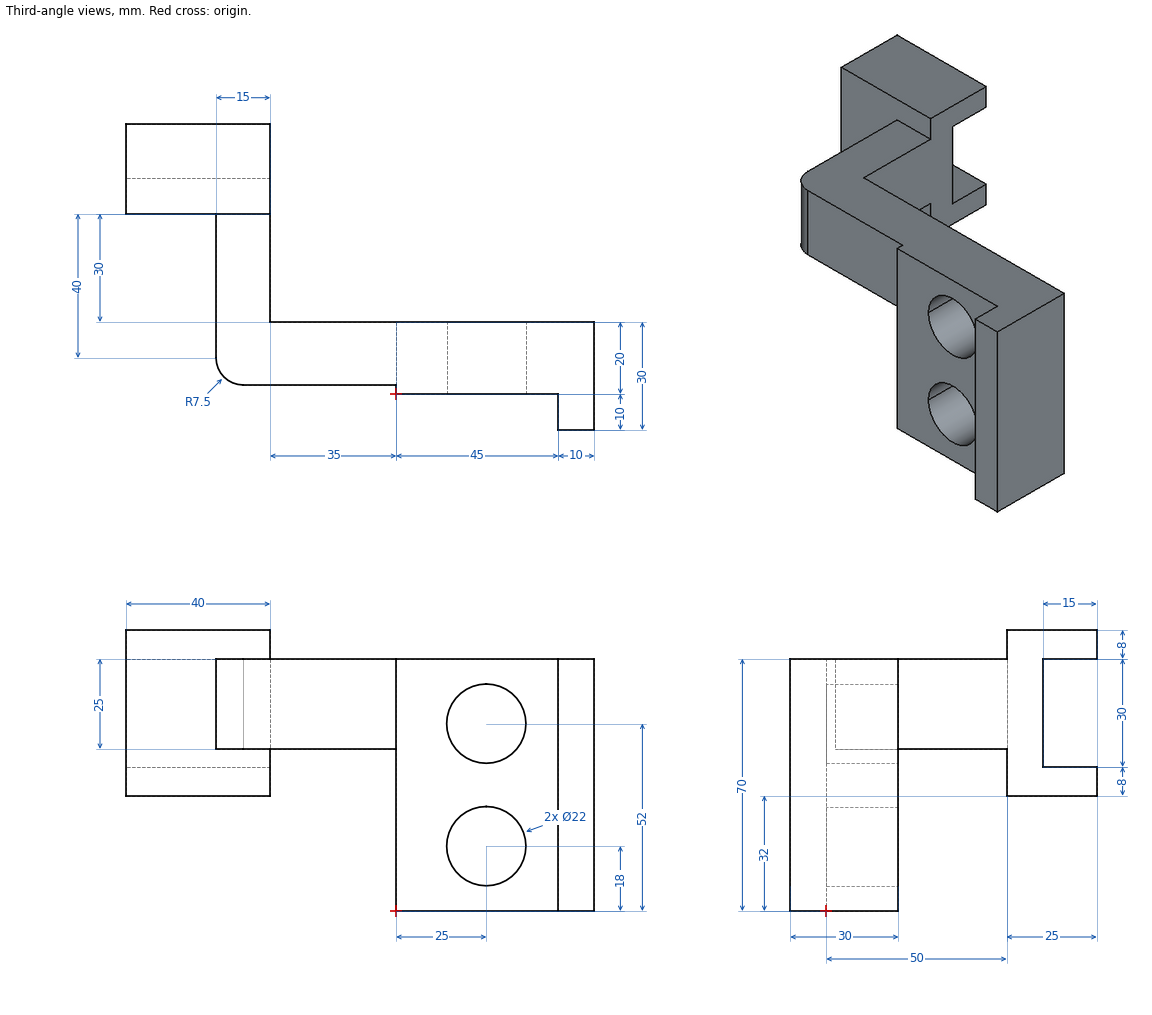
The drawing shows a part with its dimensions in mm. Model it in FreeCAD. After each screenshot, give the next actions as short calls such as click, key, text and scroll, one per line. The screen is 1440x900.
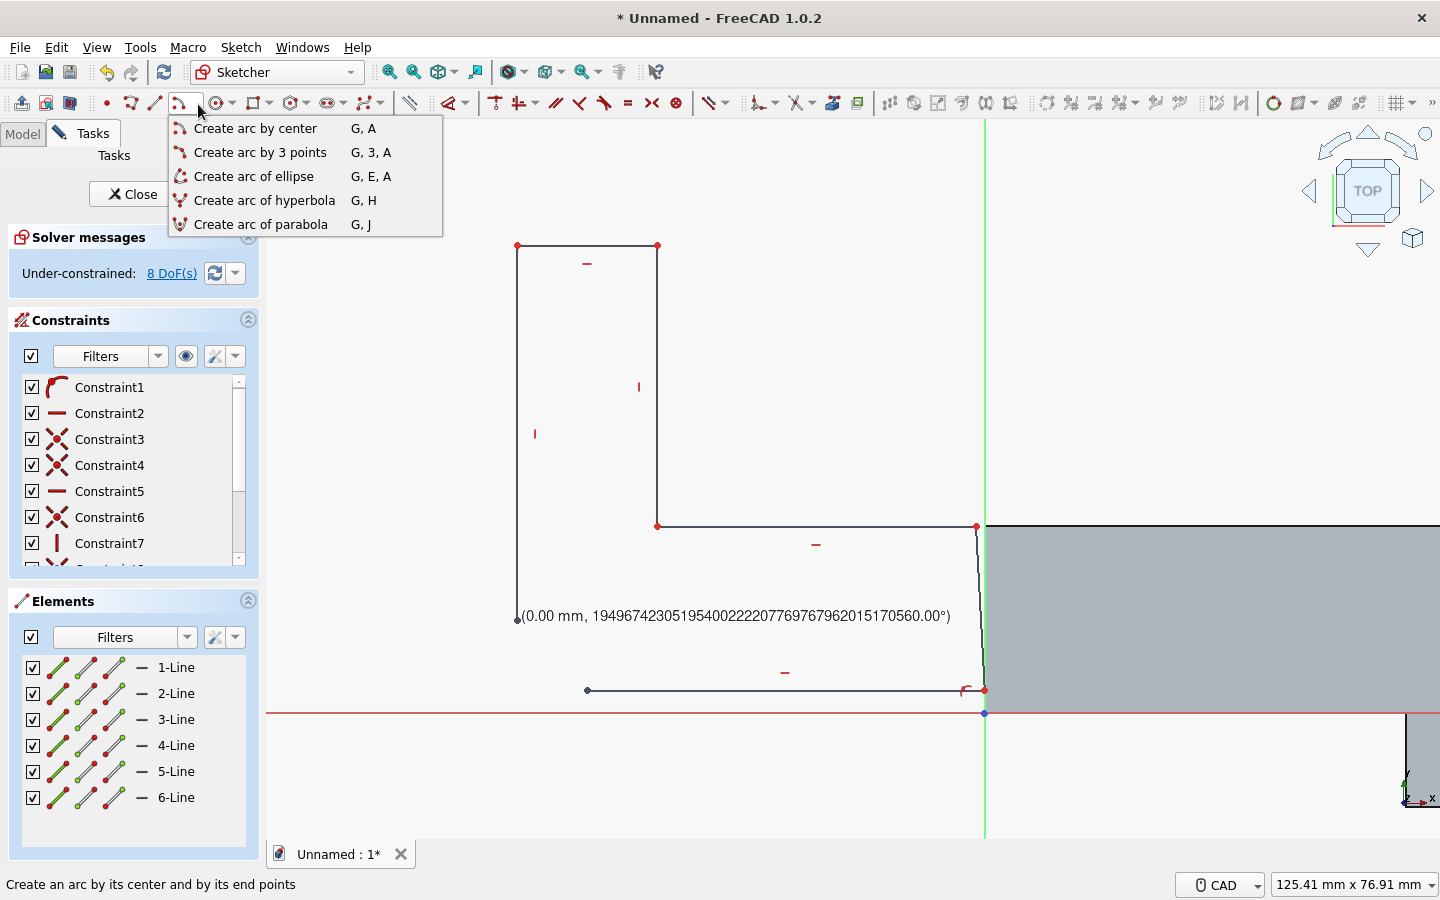
click(306, 152)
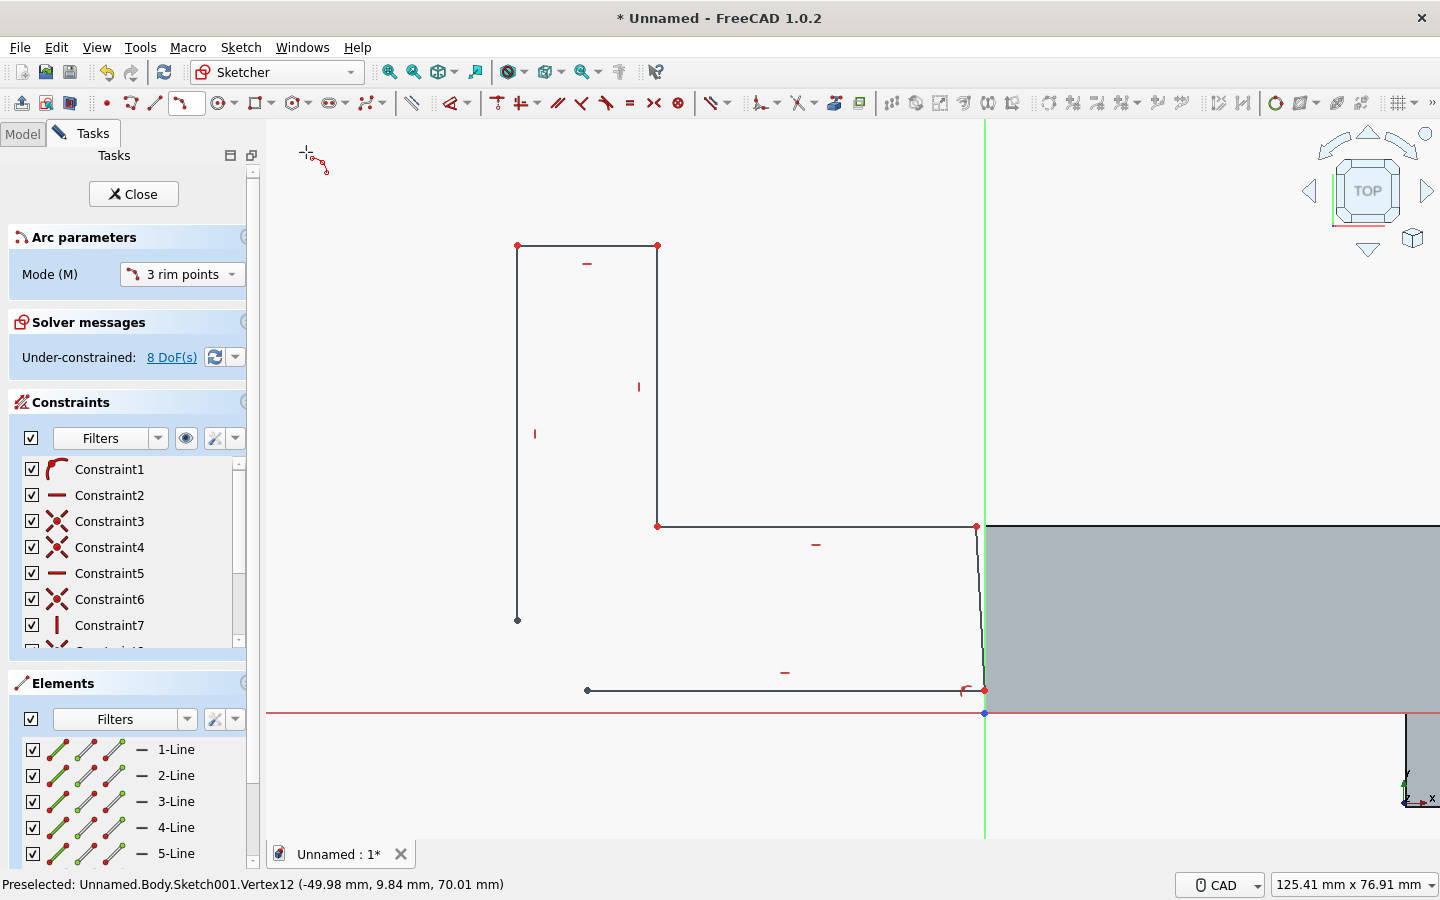
click(517, 621)
click(587, 691)
click(537, 669)
key(Escape)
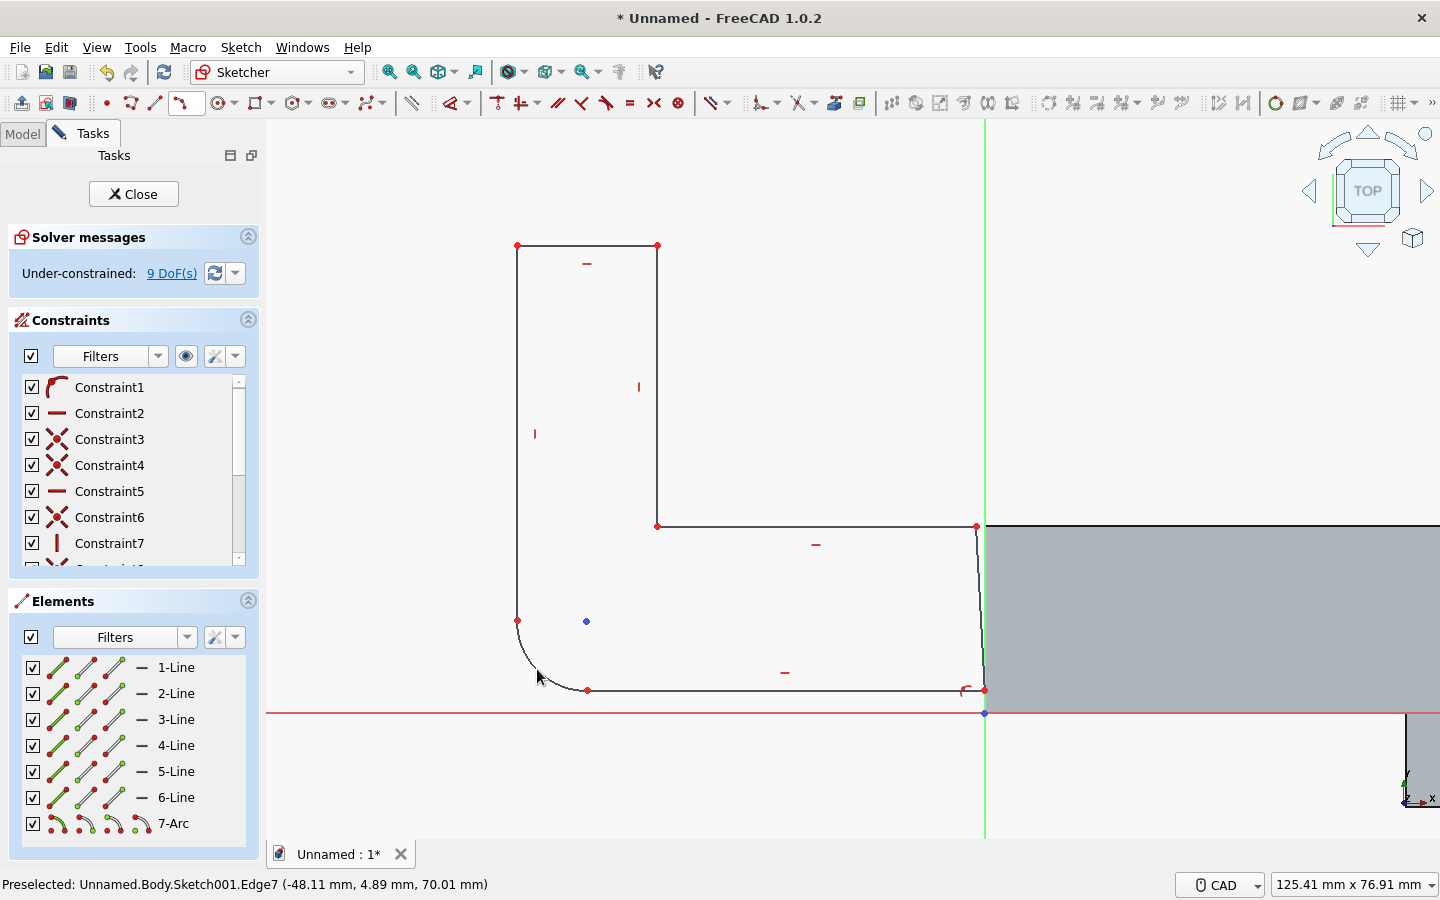
click(706, 691)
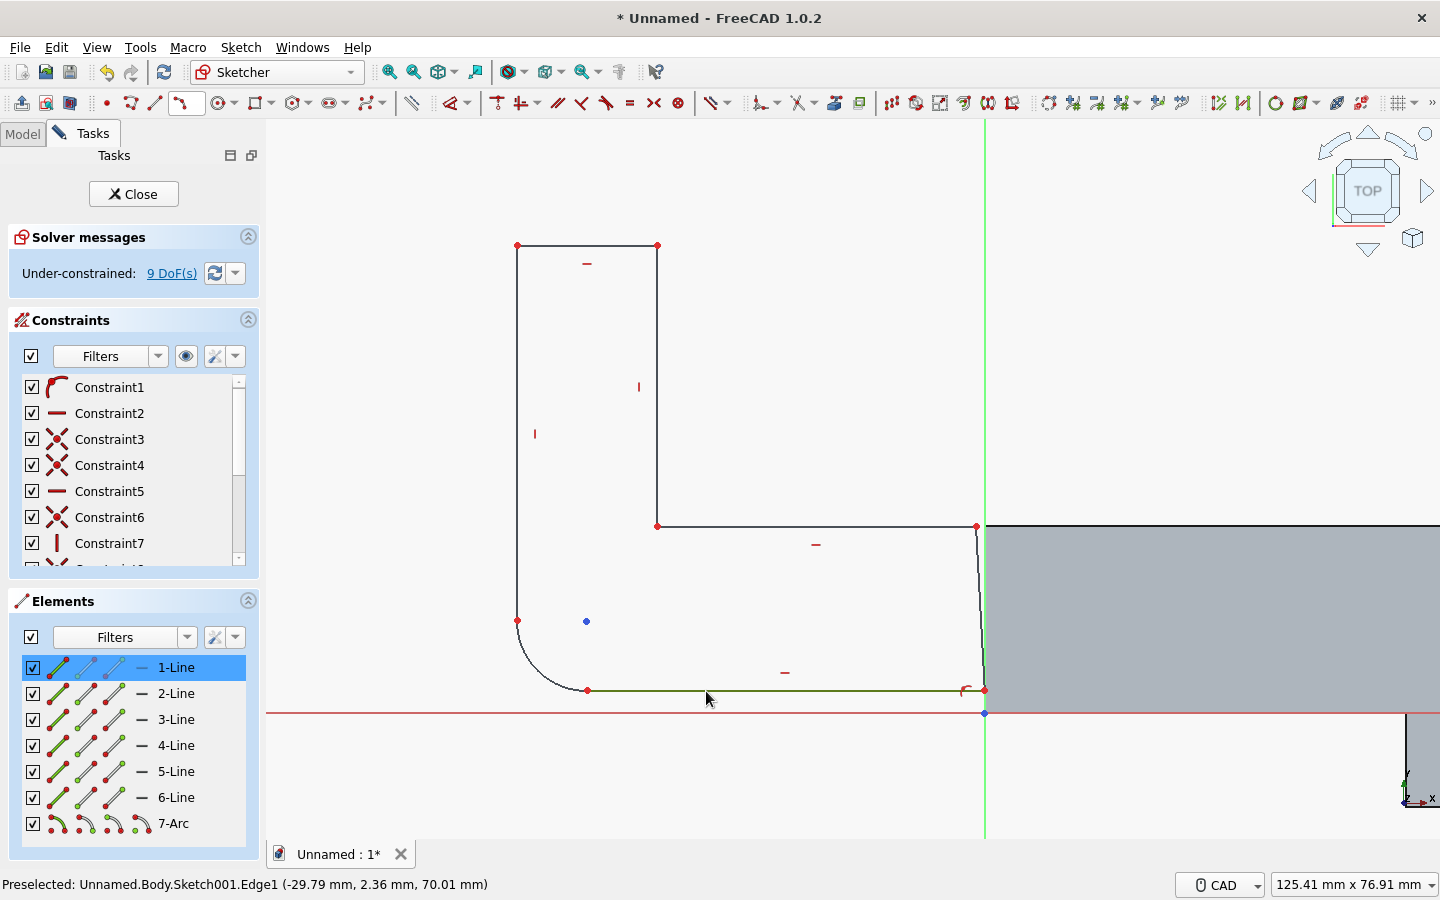
click(525, 653)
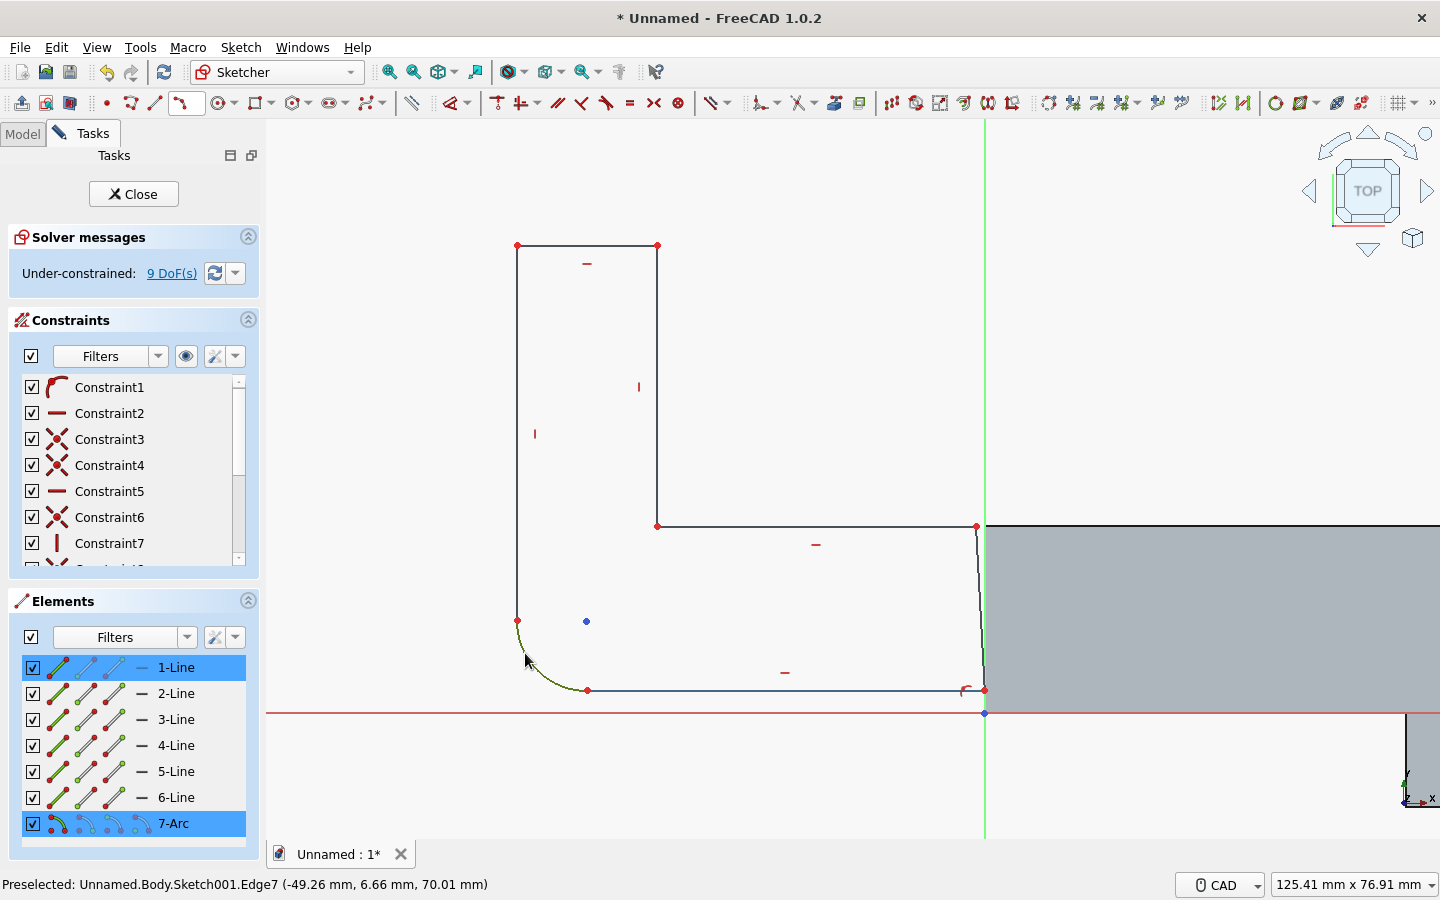
key(t)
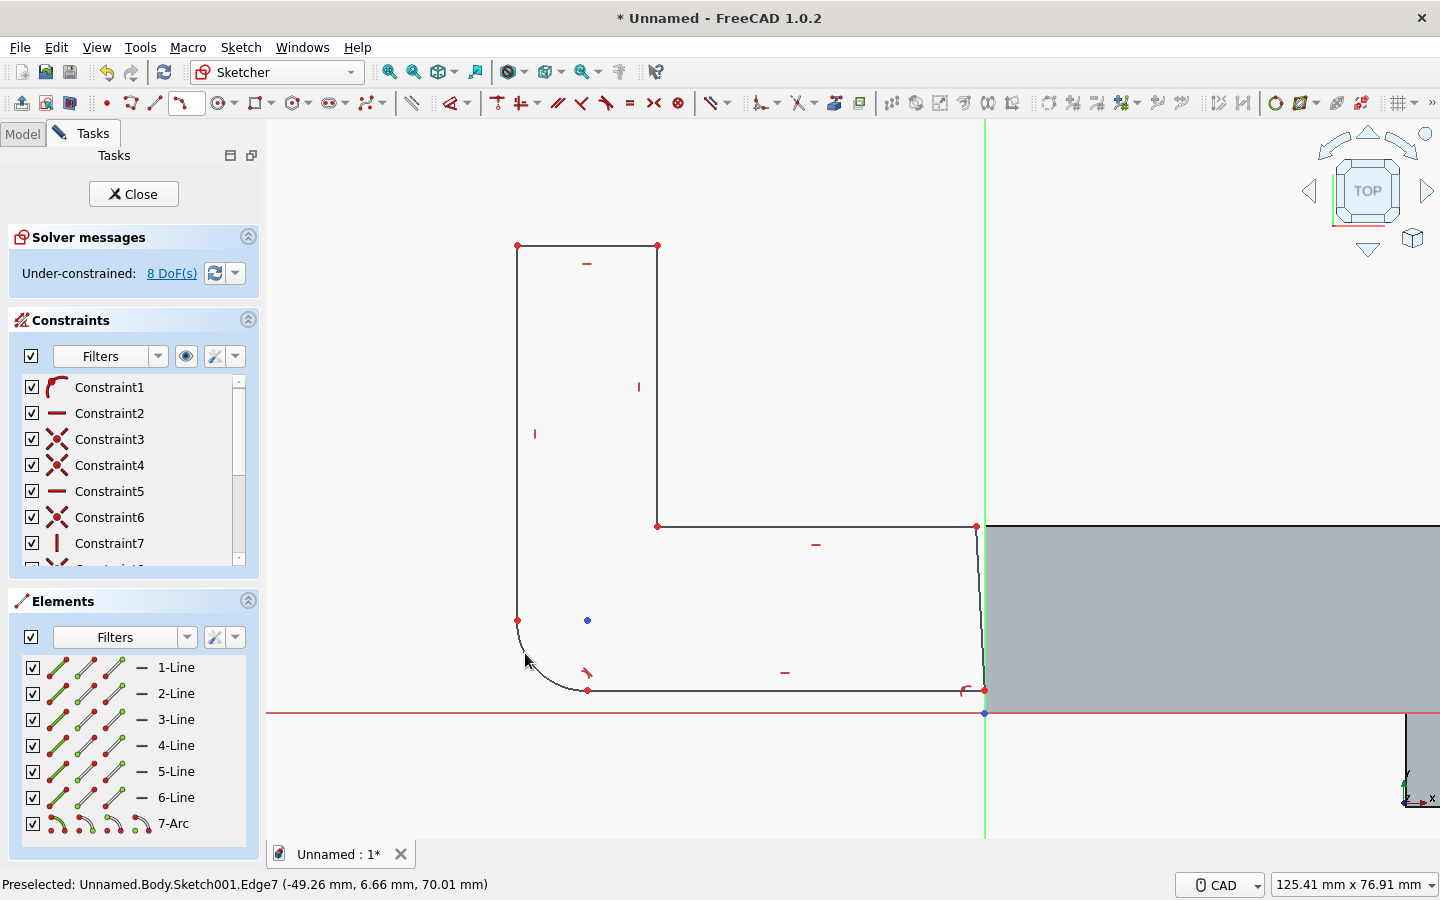
click(517, 359)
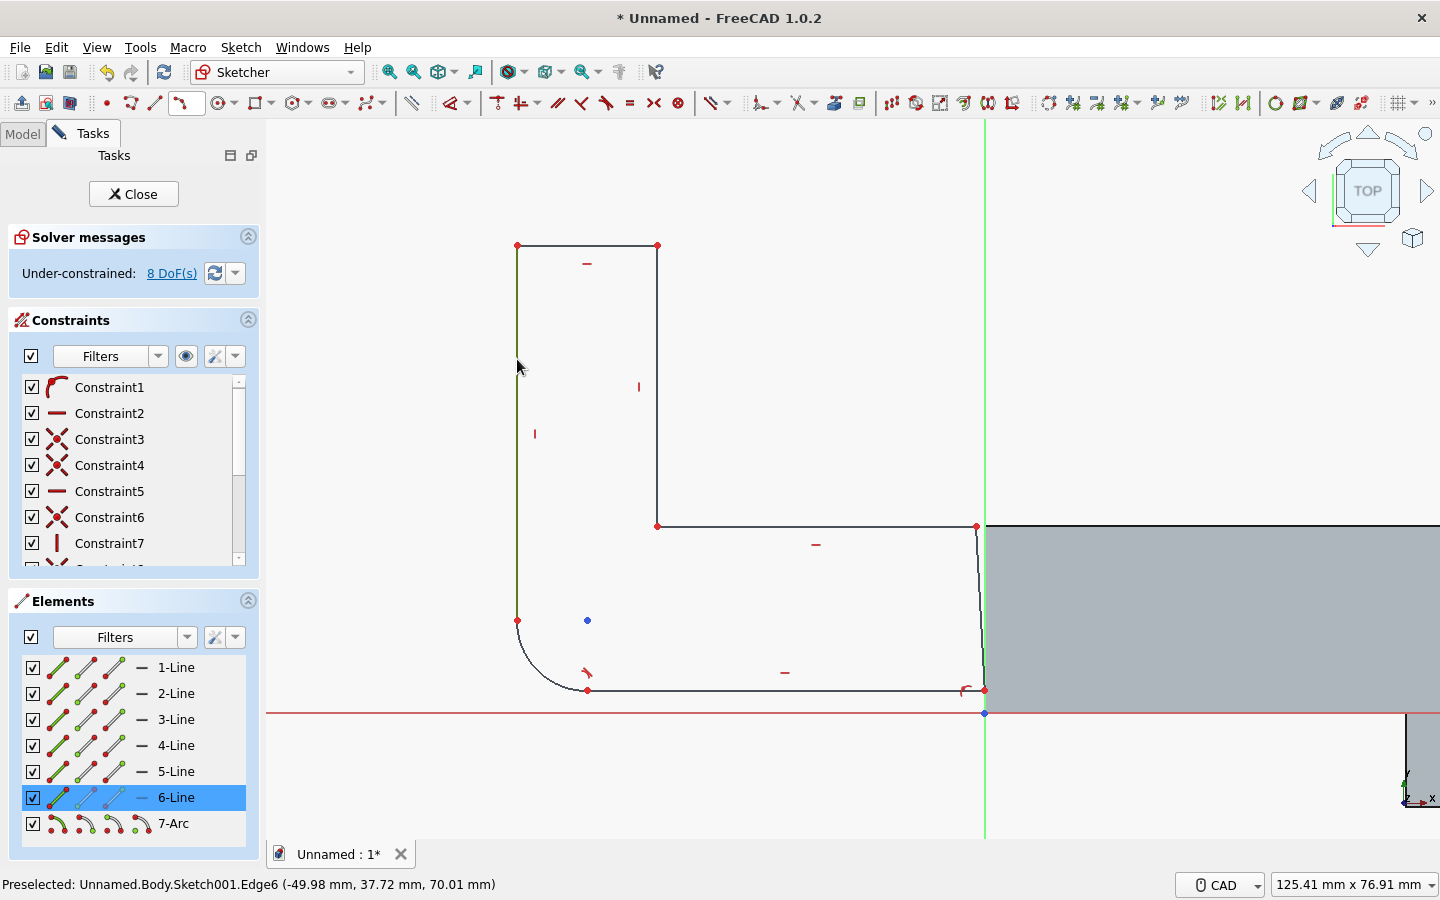
click(525, 653)